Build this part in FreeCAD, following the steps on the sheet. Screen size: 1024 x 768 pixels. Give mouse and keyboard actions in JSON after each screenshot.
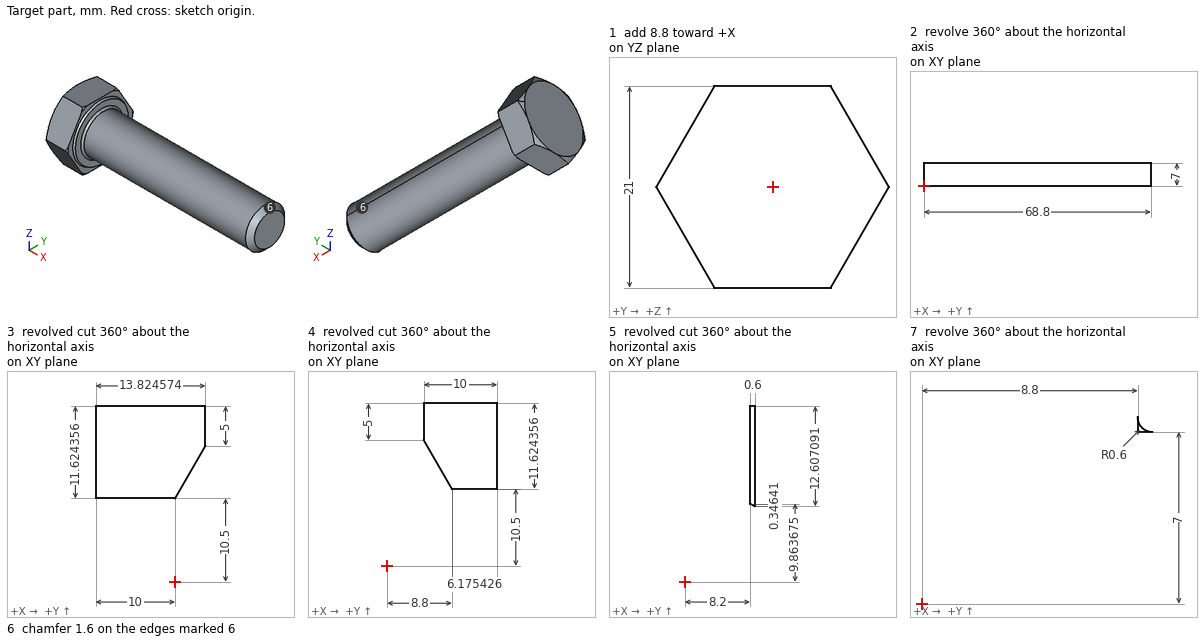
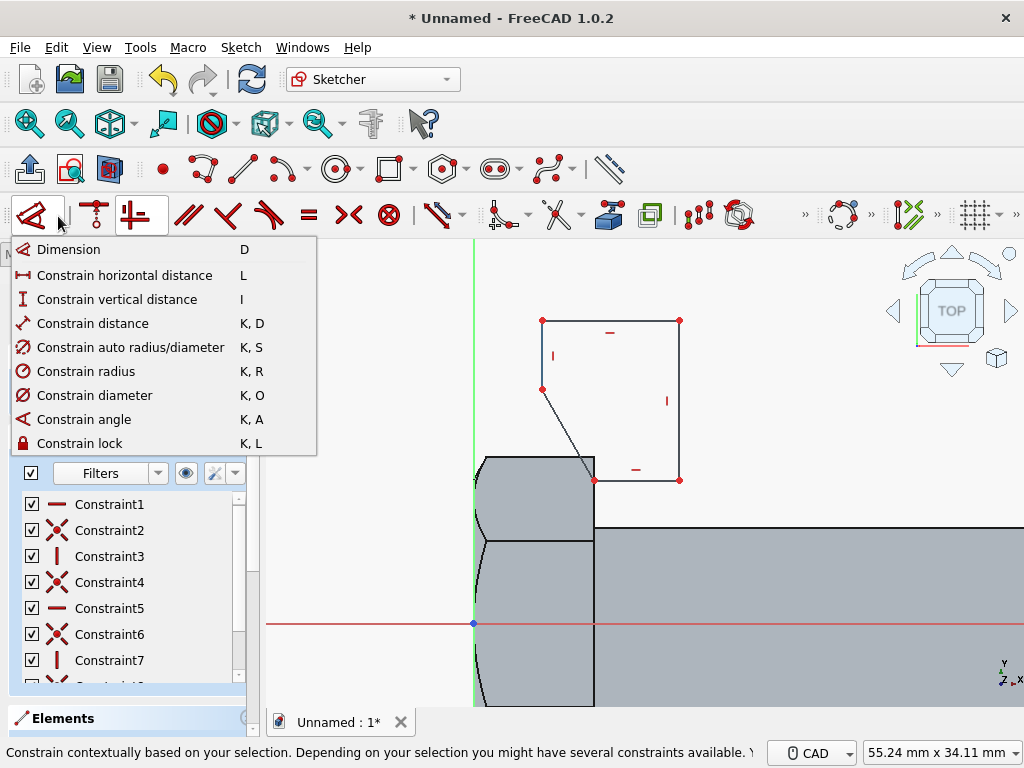
{"action": "left_click", "coordinate": [164, 299]}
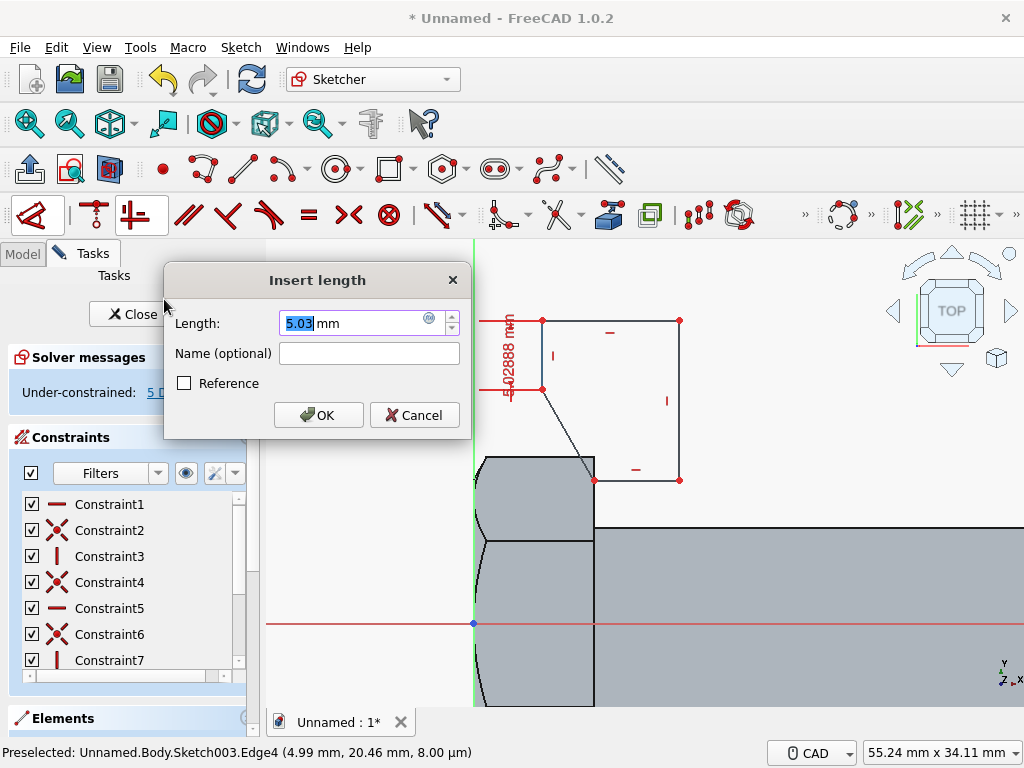
{"action": "type", "text": "5"}
{"action": "key", "text": "Return"}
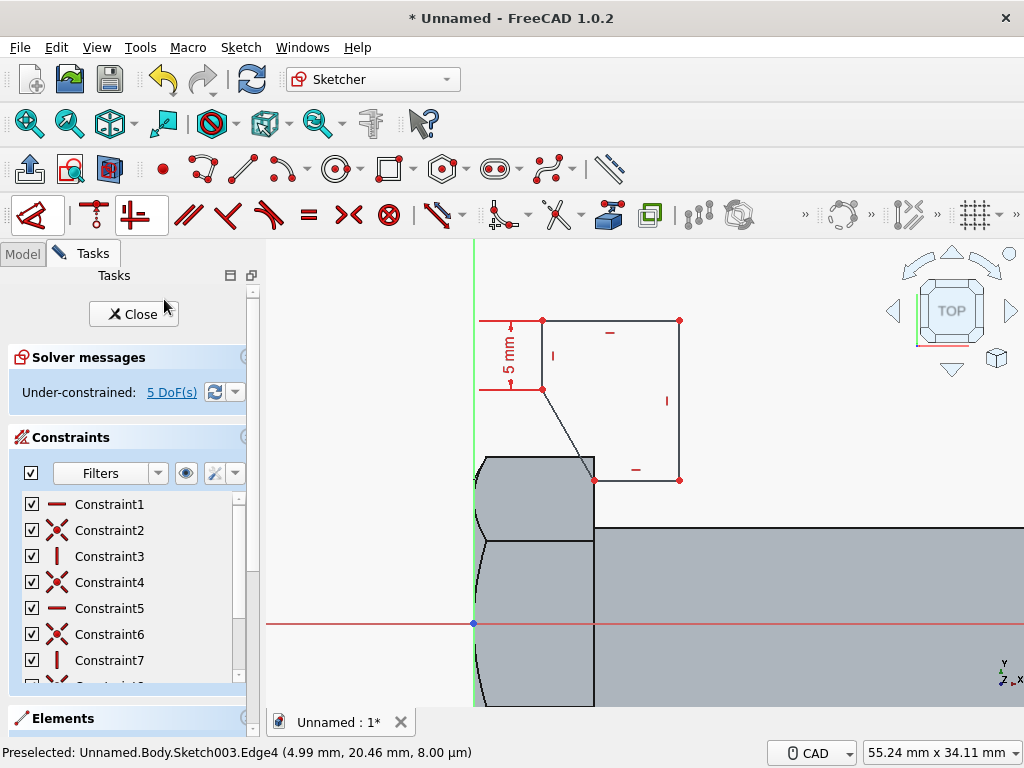
{"action": "left_click", "coordinate": [638, 321]}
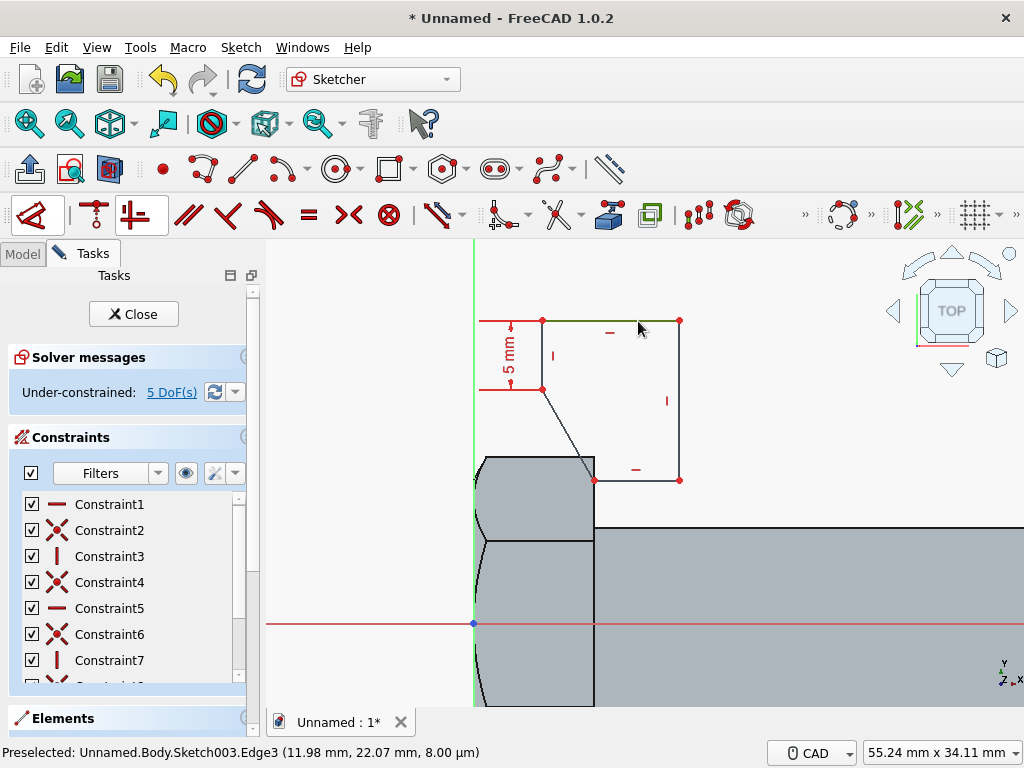
{"action": "key", "text": "l"}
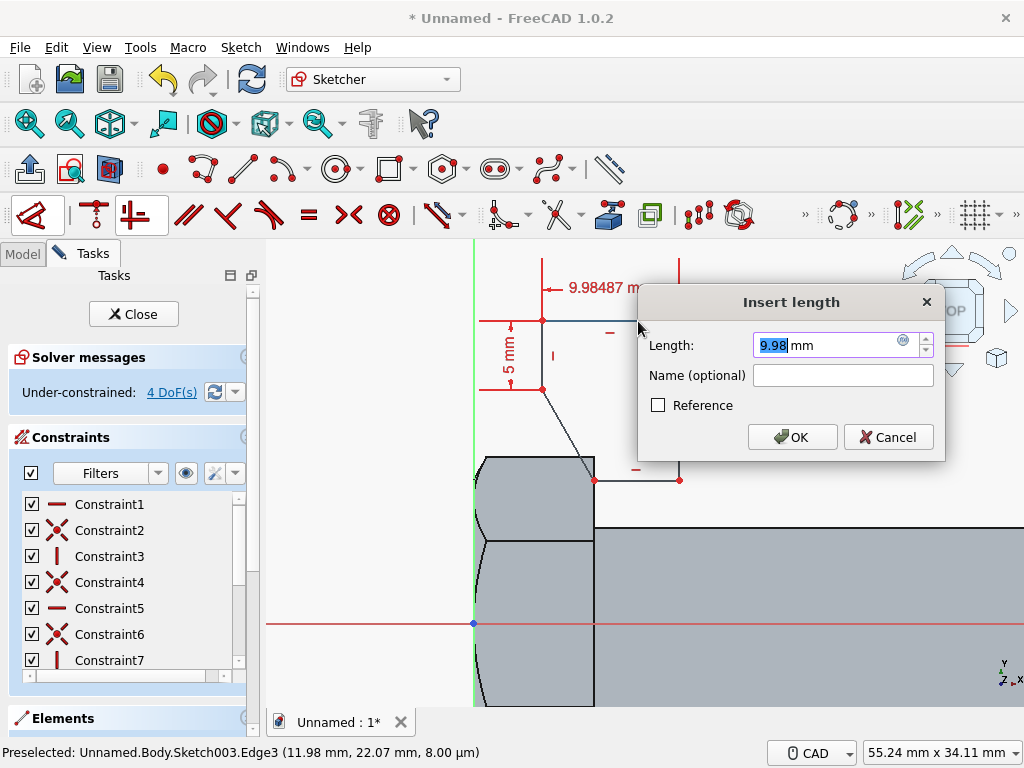
{"action": "type", "text": "10"}
{"action": "key", "text": "Return"}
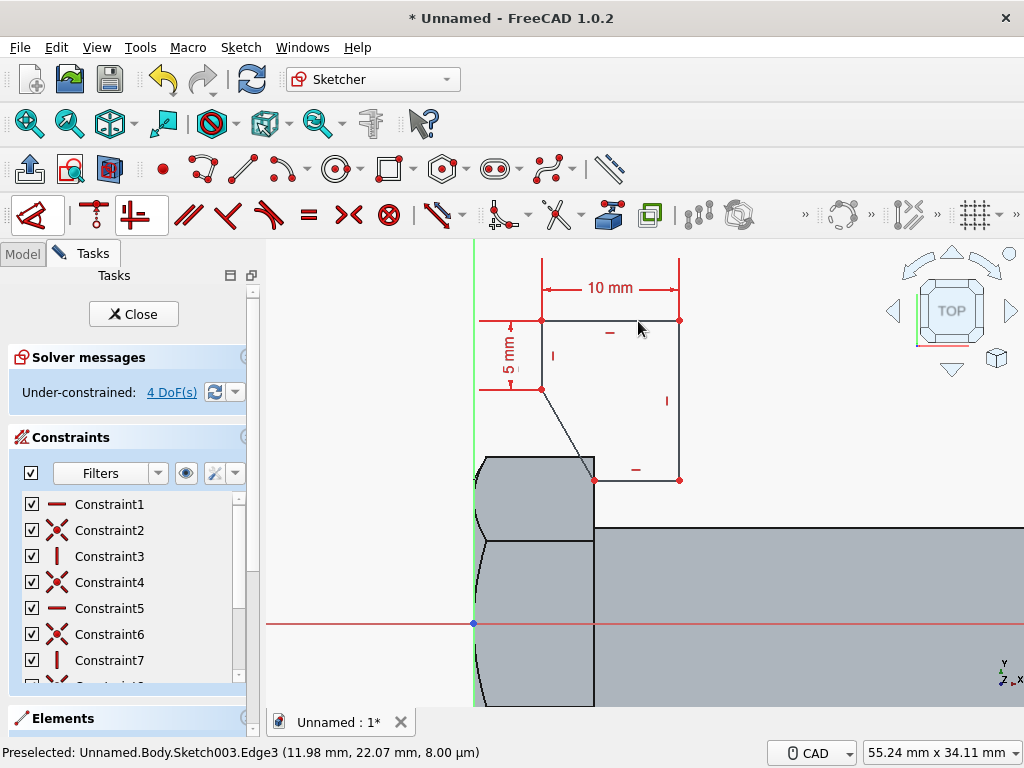
{"action": "left_click", "coordinate": [594, 481]}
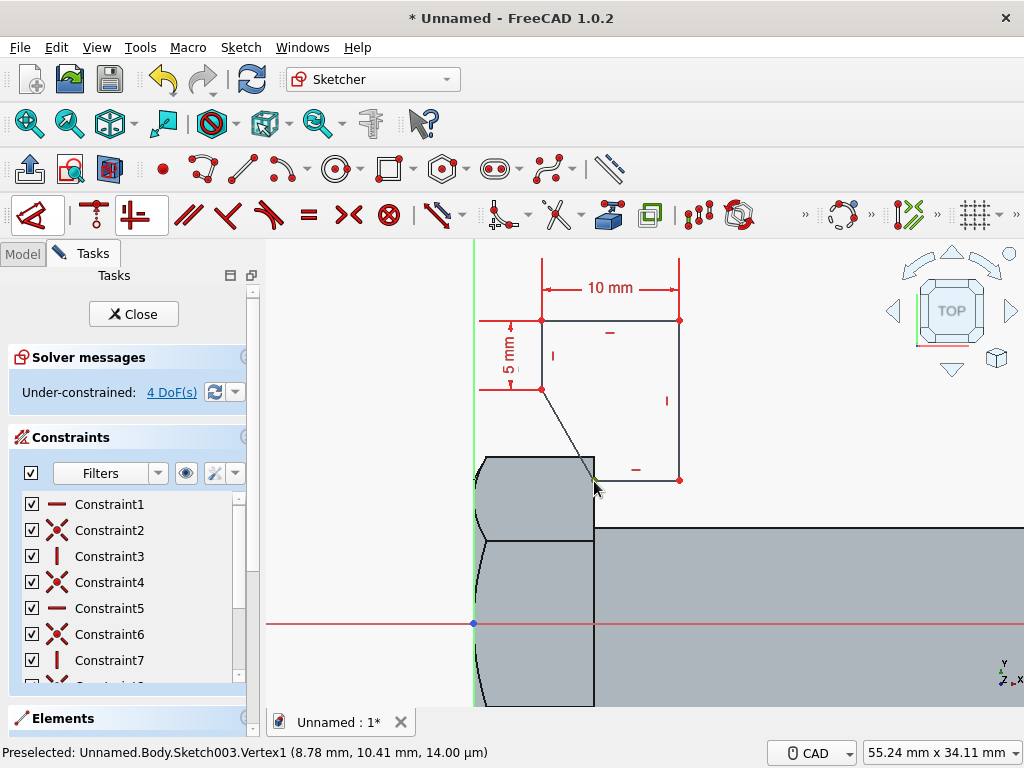
{"action": "left_click", "coordinate": [58, 216]}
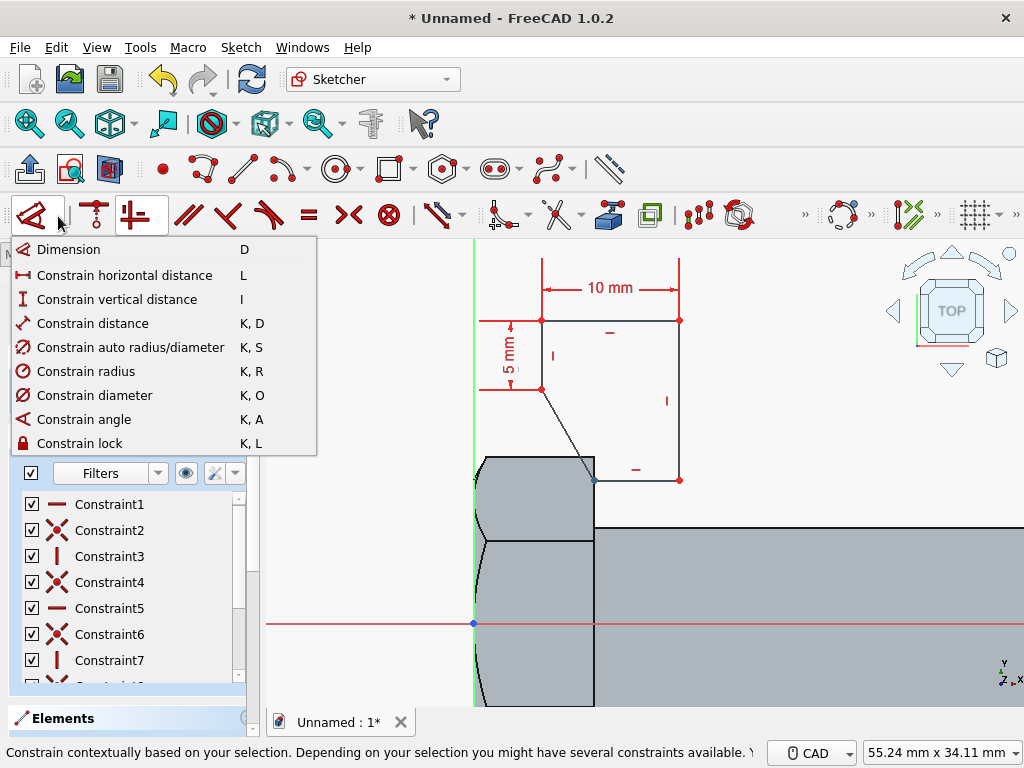
{"action": "left_click", "coordinate": [164, 275]}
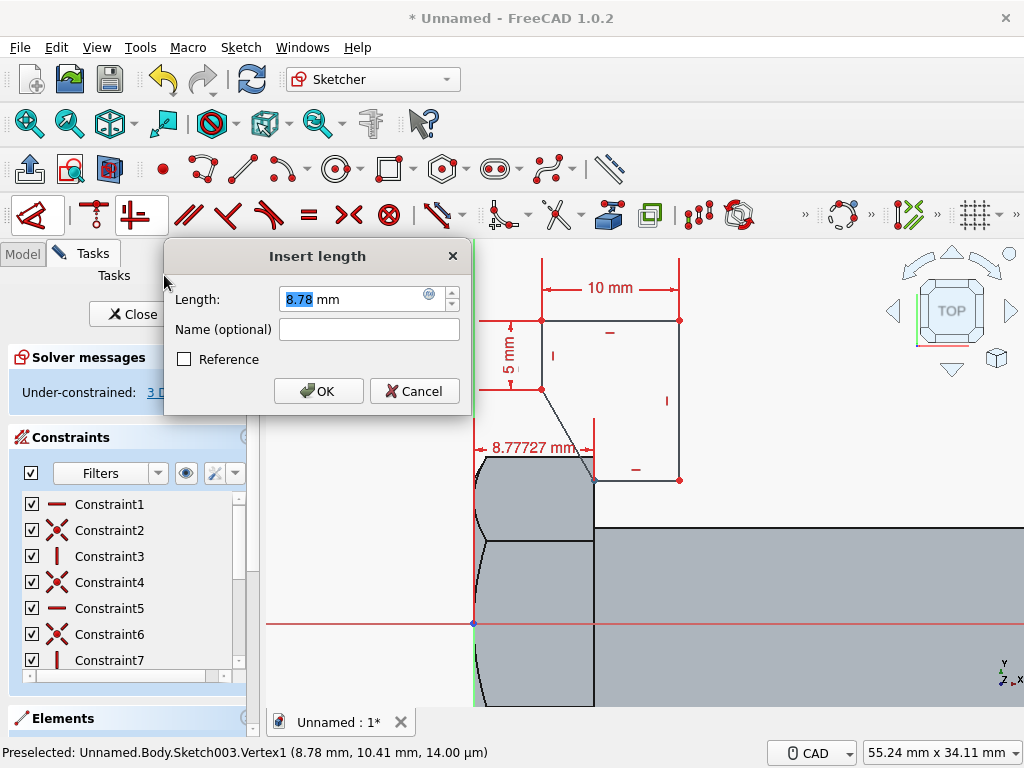
{"action": "type", "text": "8.8"}
{"action": "key", "text": "Return"}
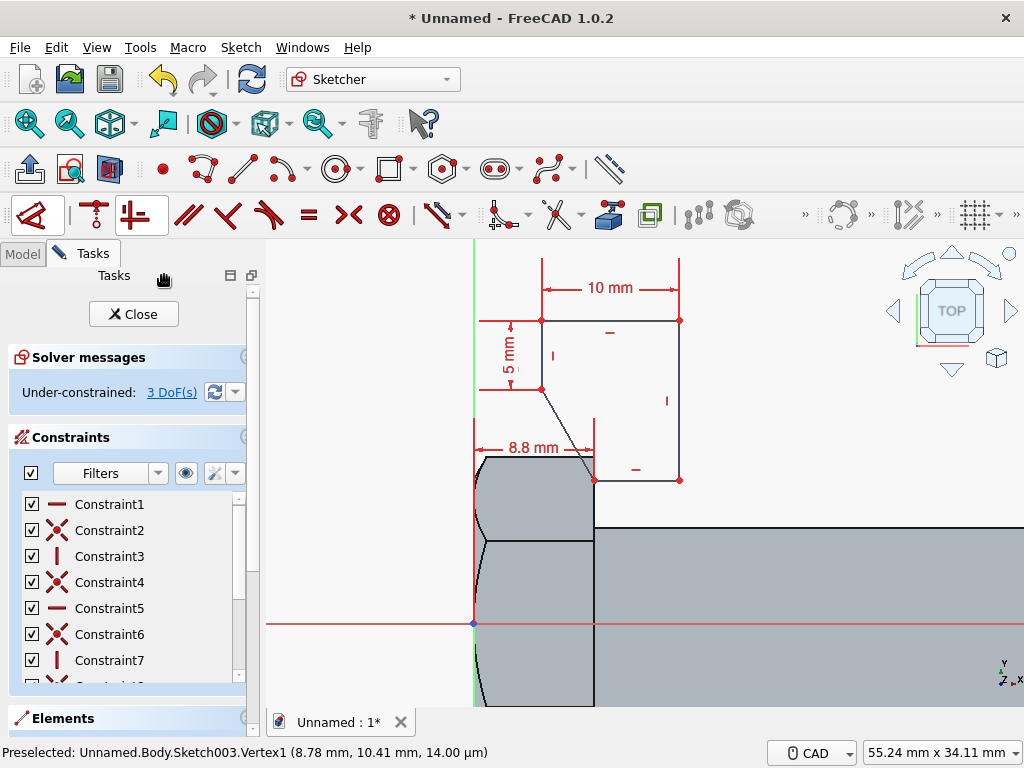
{"action": "left_click", "coordinate": [594, 481]}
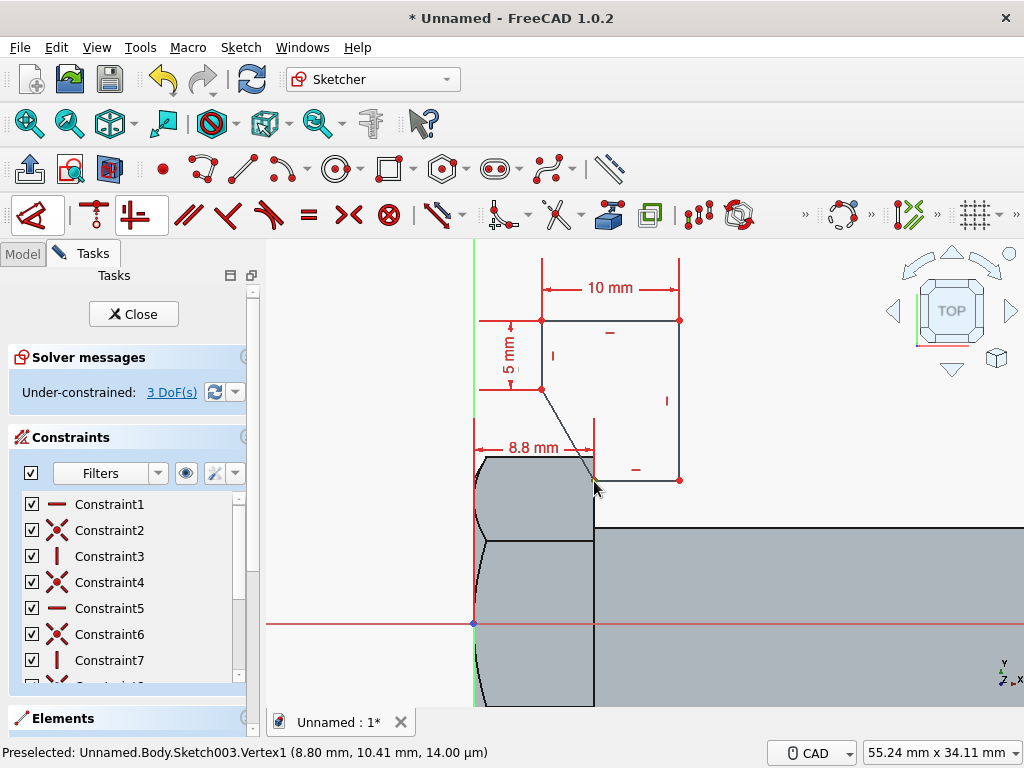
{"action": "left_click", "coordinate": [58, 216]}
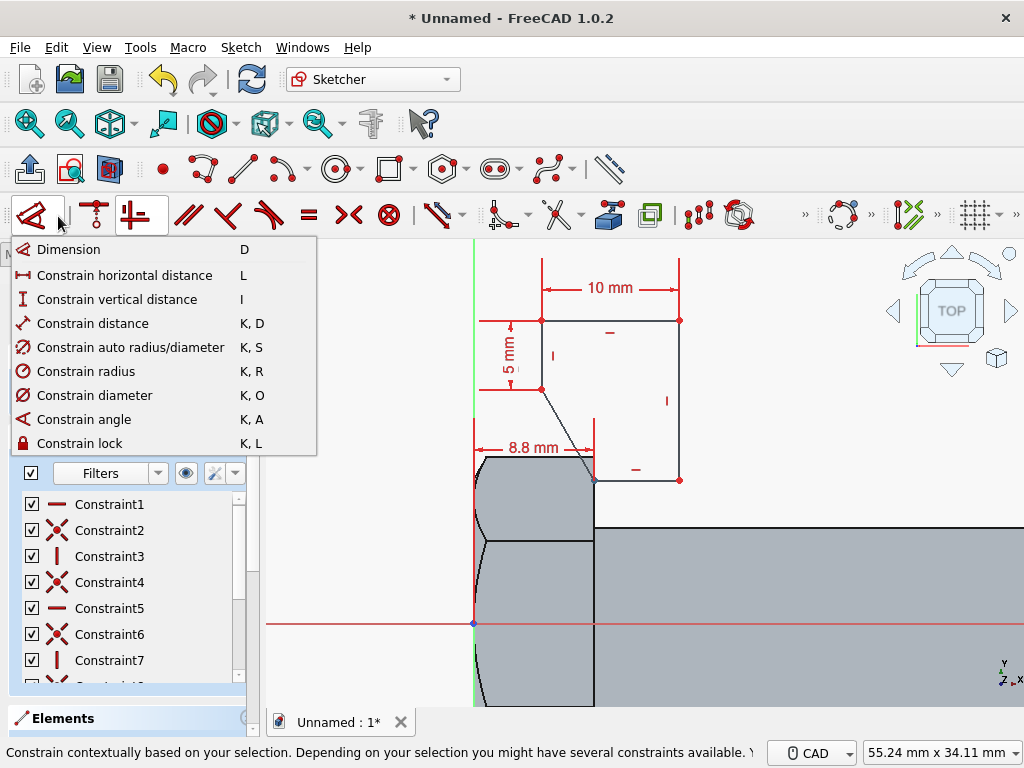
{"action": "left_click", "coordinate": [164, 299]}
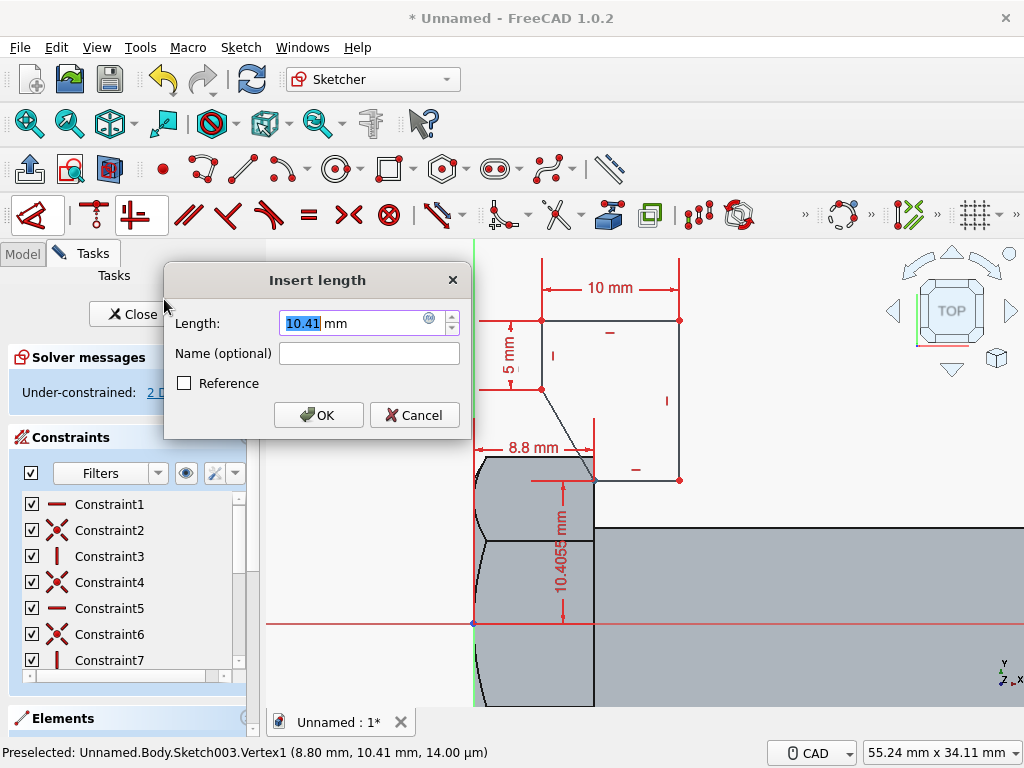
{"action": "type", "text": "10.5"}
{"action": "key", "text": "Return"}